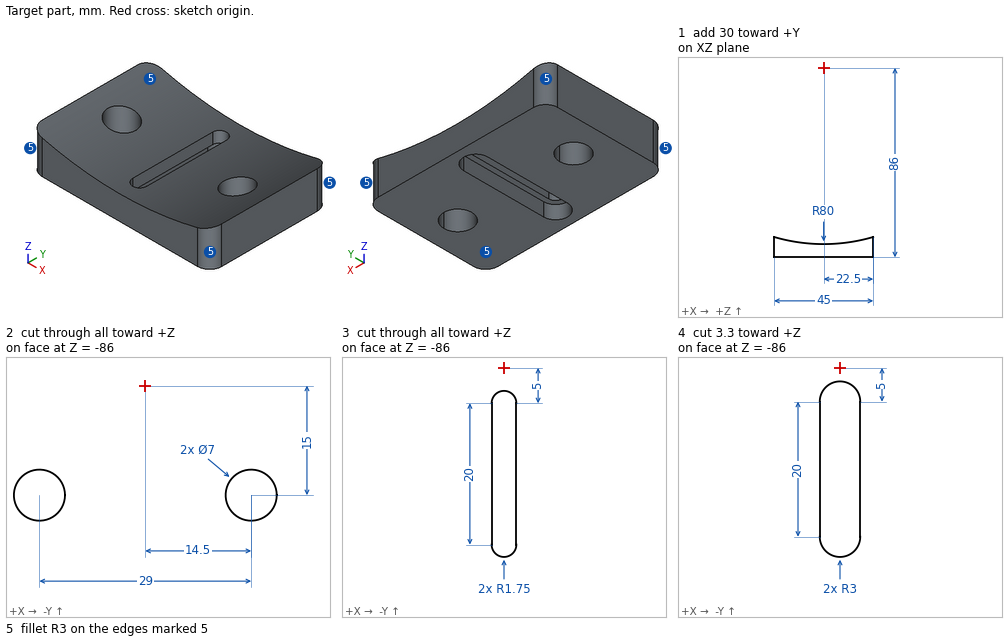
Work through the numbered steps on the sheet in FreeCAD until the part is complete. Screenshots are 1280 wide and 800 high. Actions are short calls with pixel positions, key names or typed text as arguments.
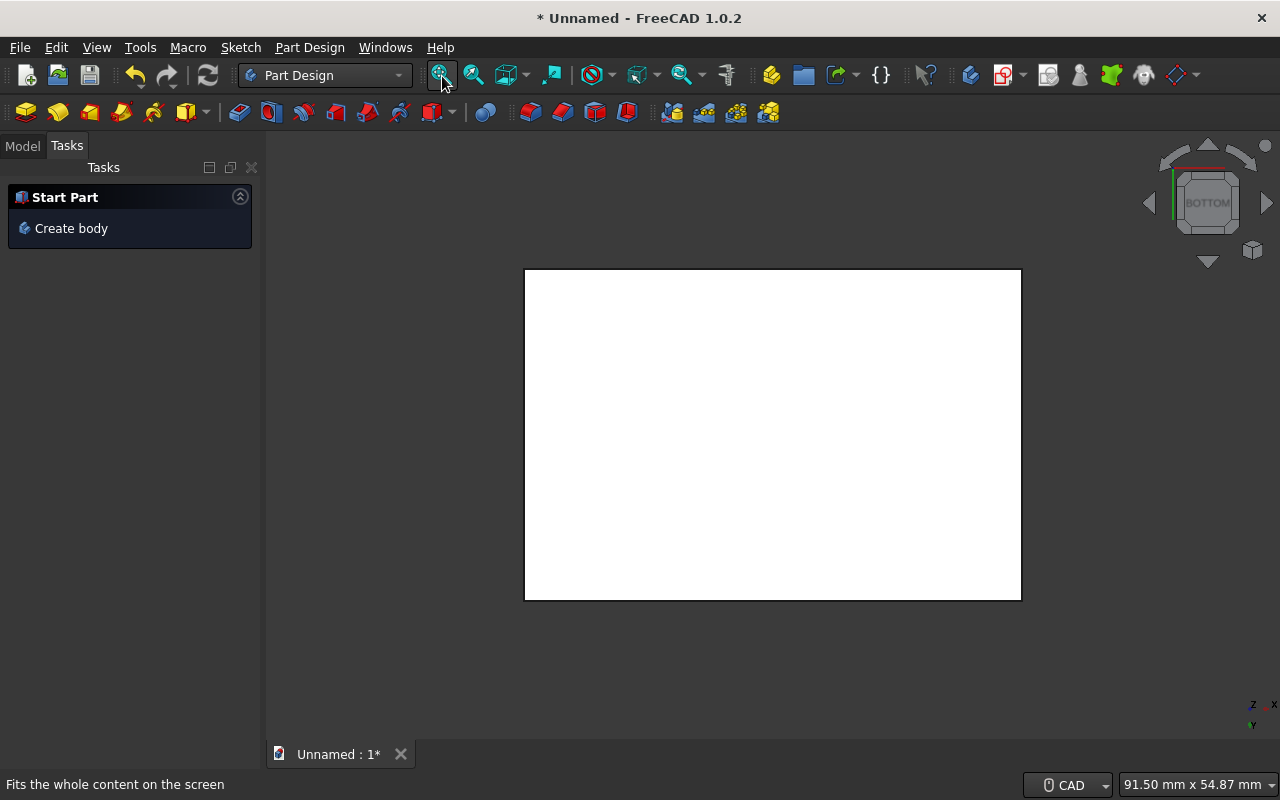
click(844, 434)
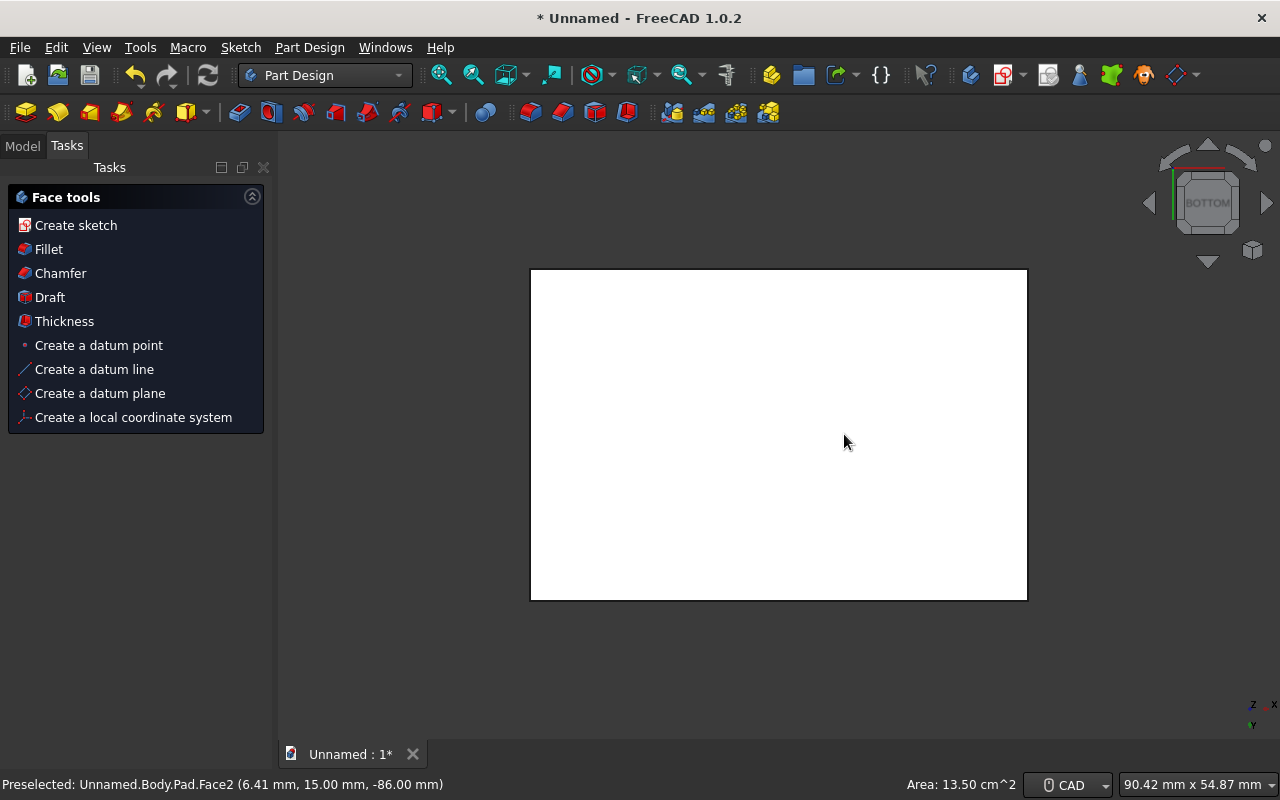
click(1004, 76)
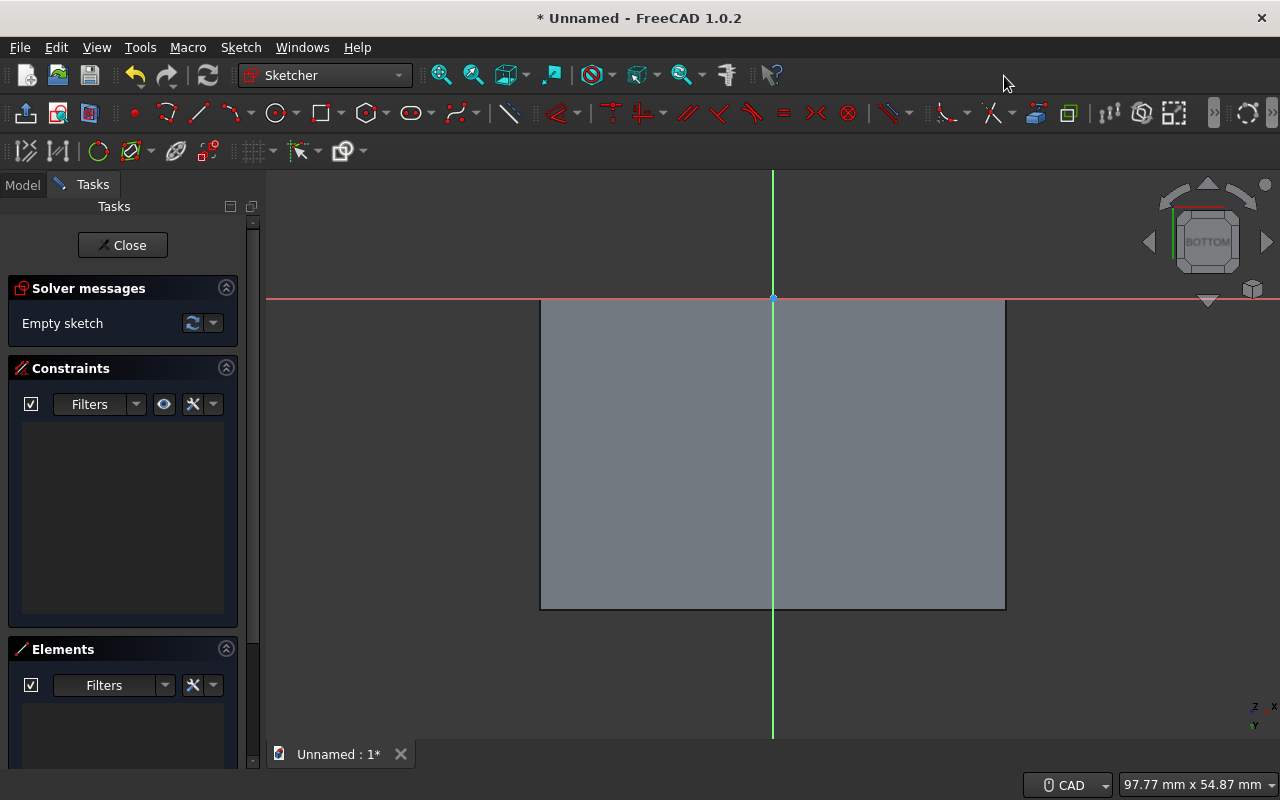
scroll(912, 274, up, 2)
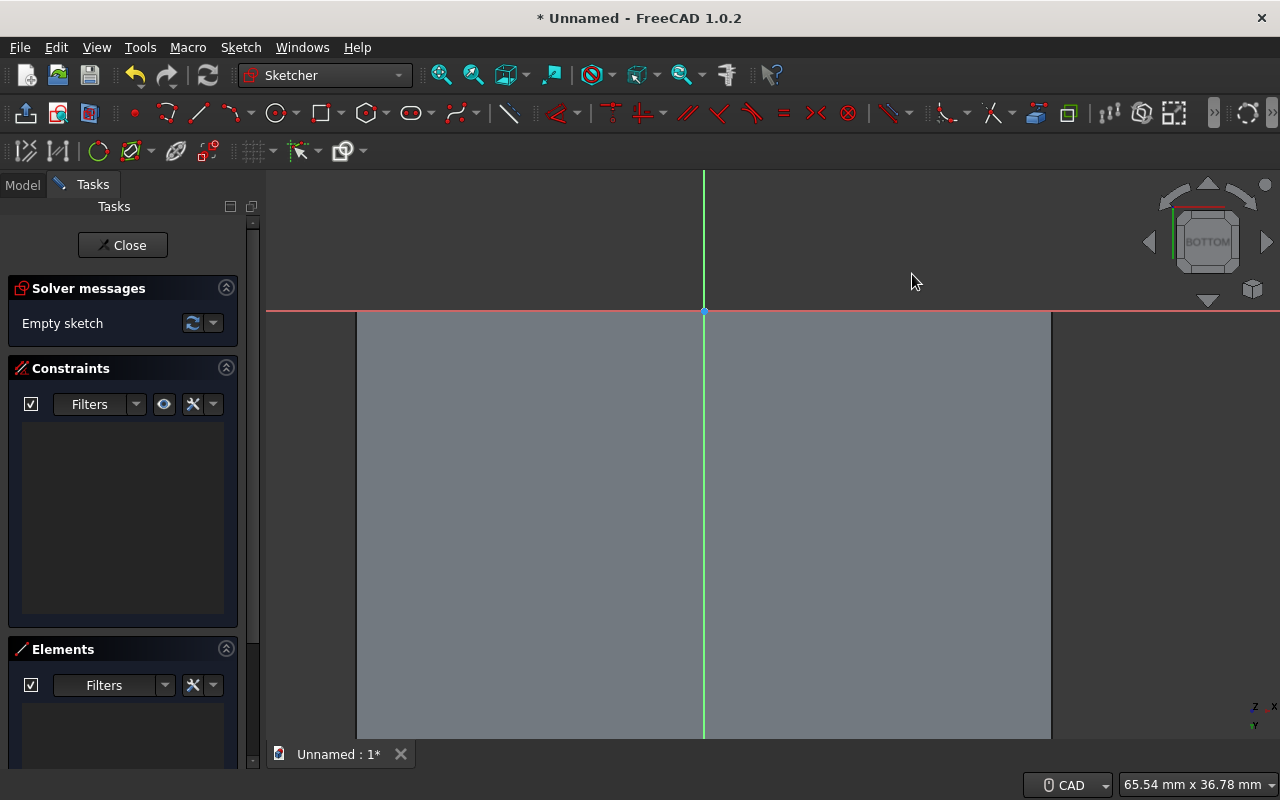
click(276, 114)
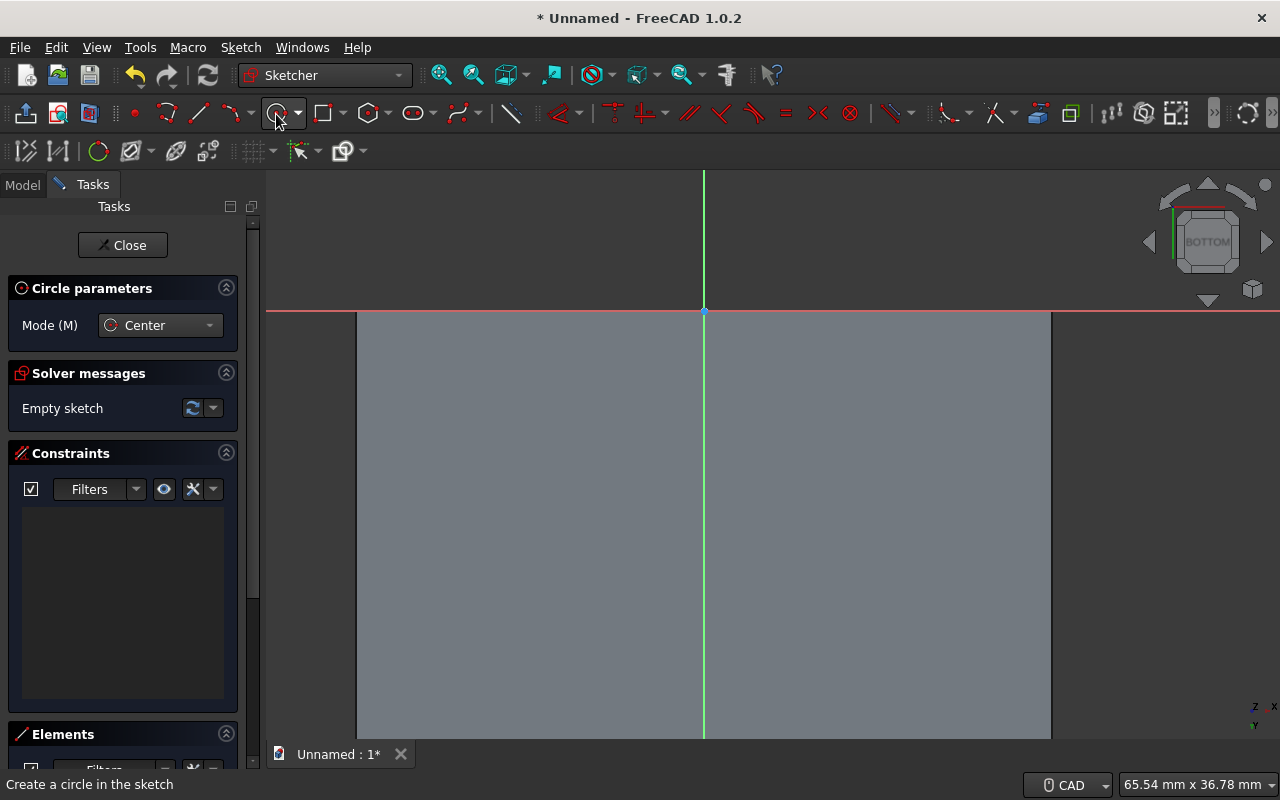
click(929, 543)
move(967, 505)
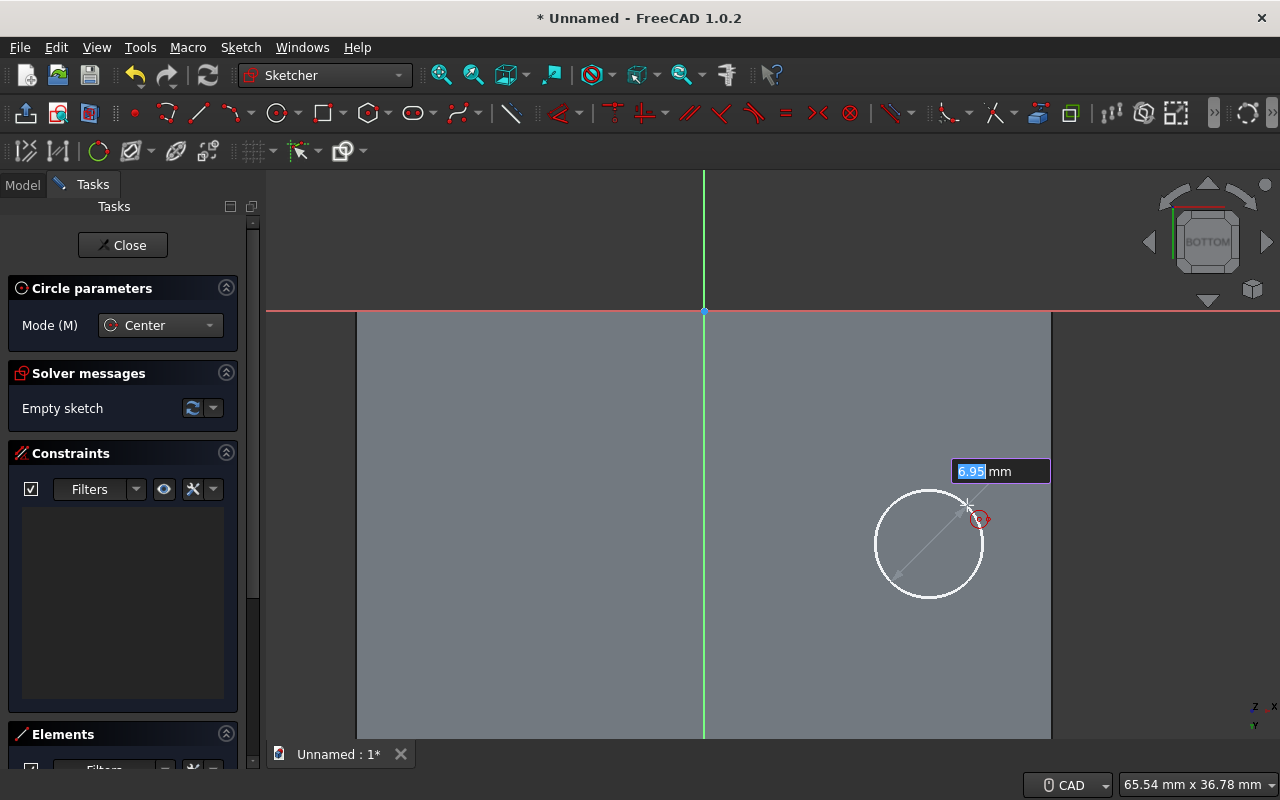
text(7)
key(Return)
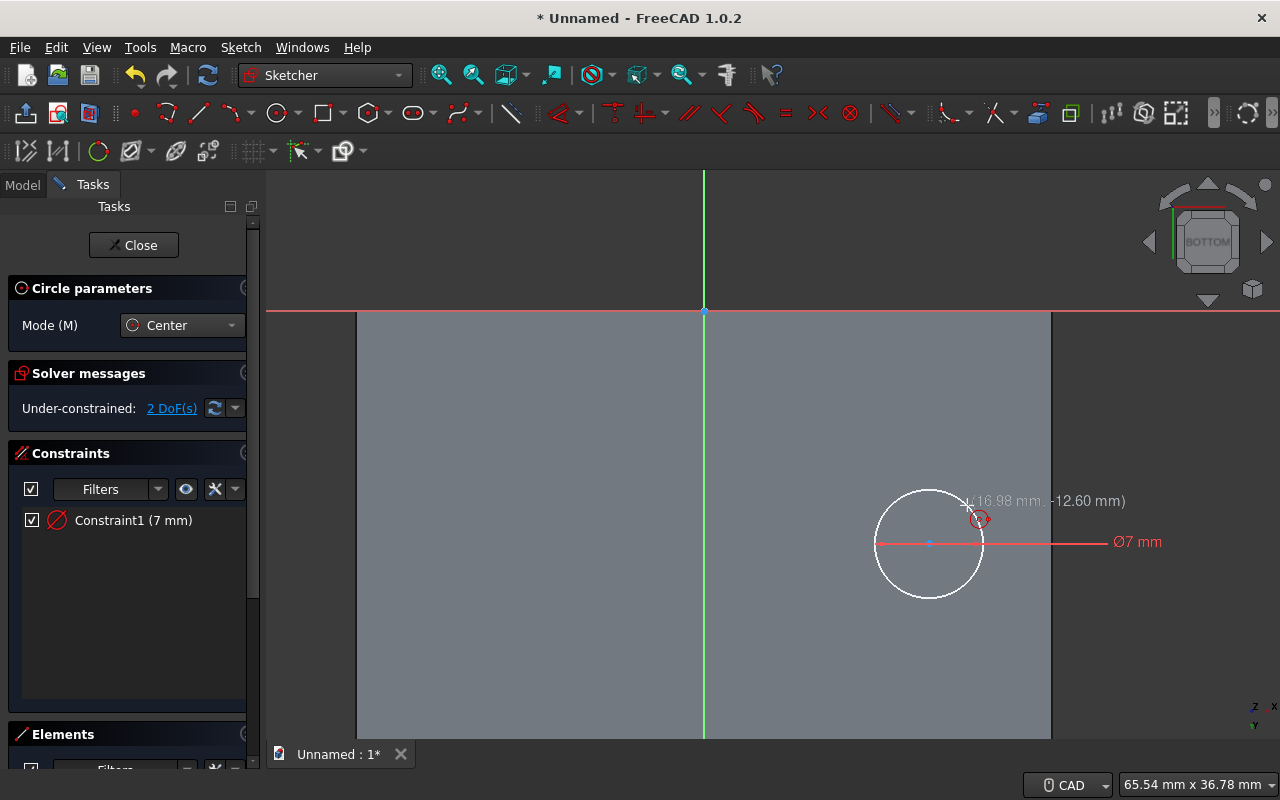
click(480, 543)
move(518, 505)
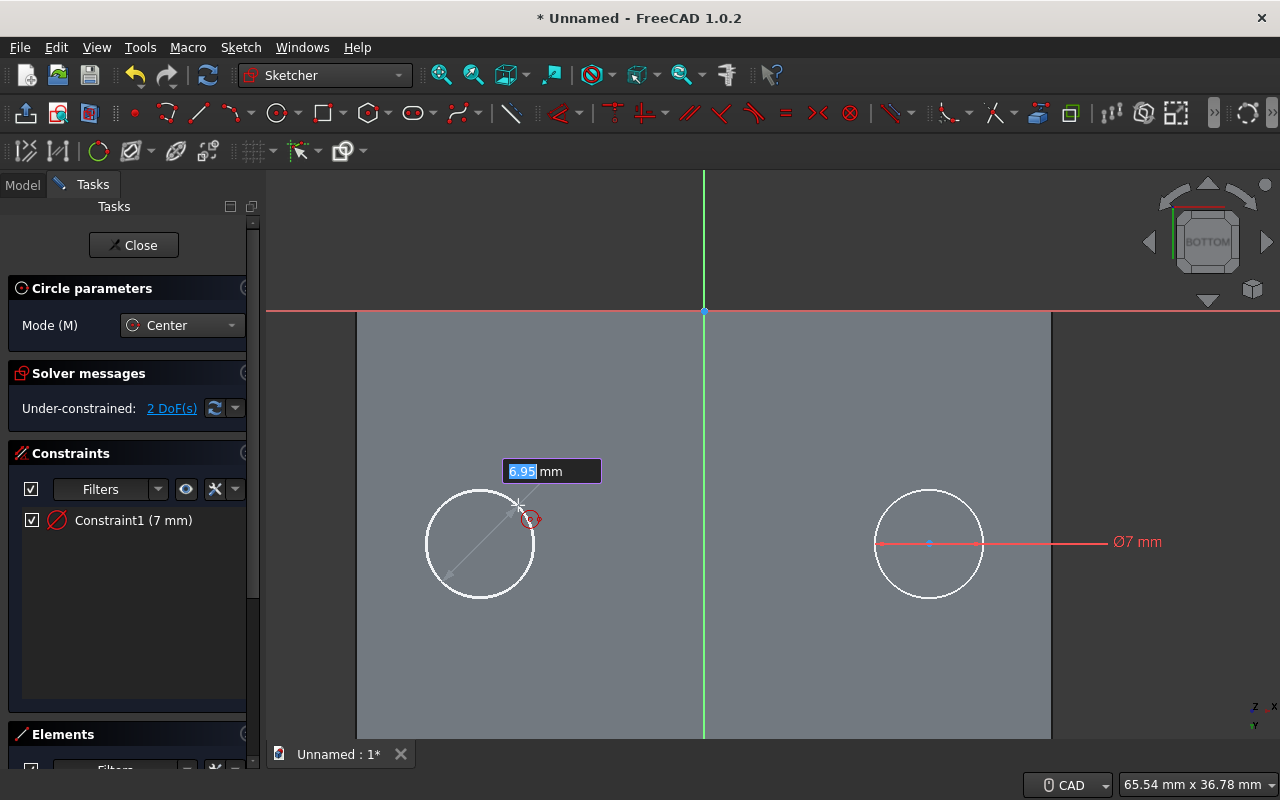
text(7)
key(Return)
key(Escape)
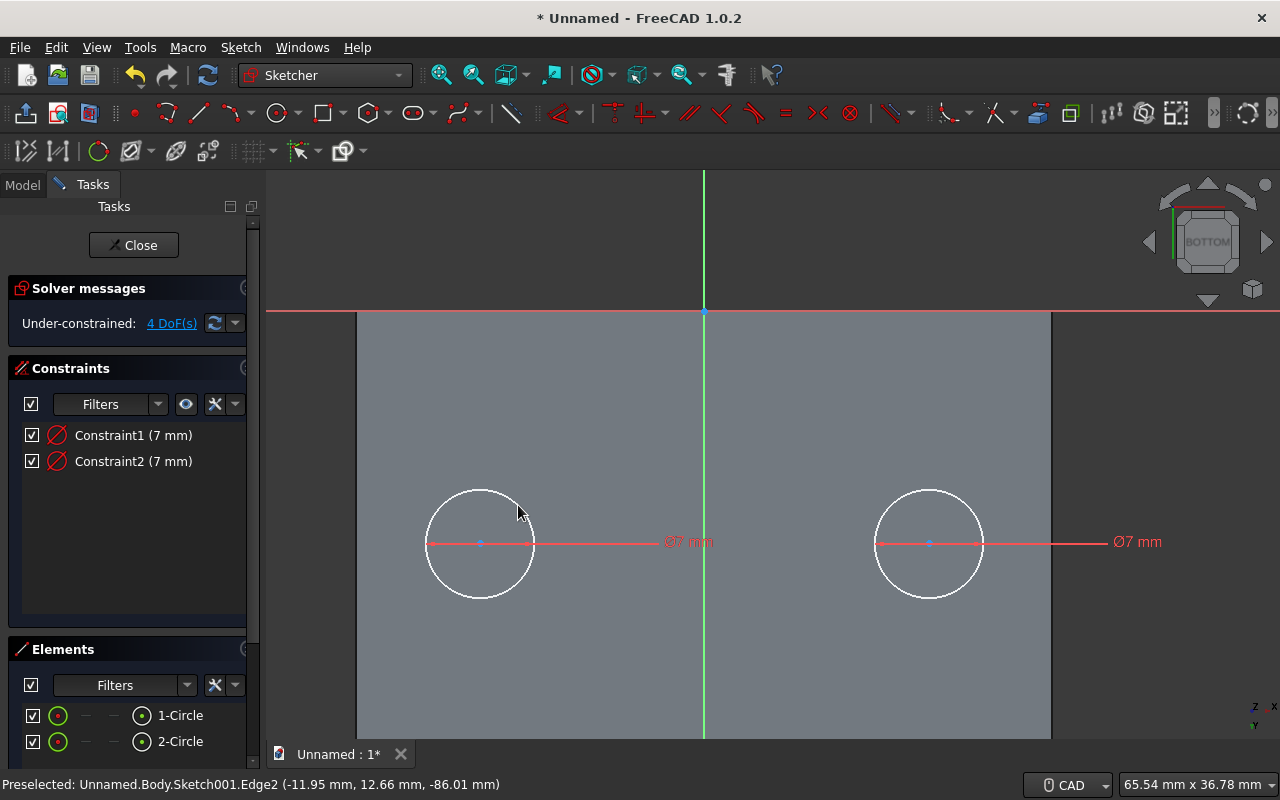
click(929, 544)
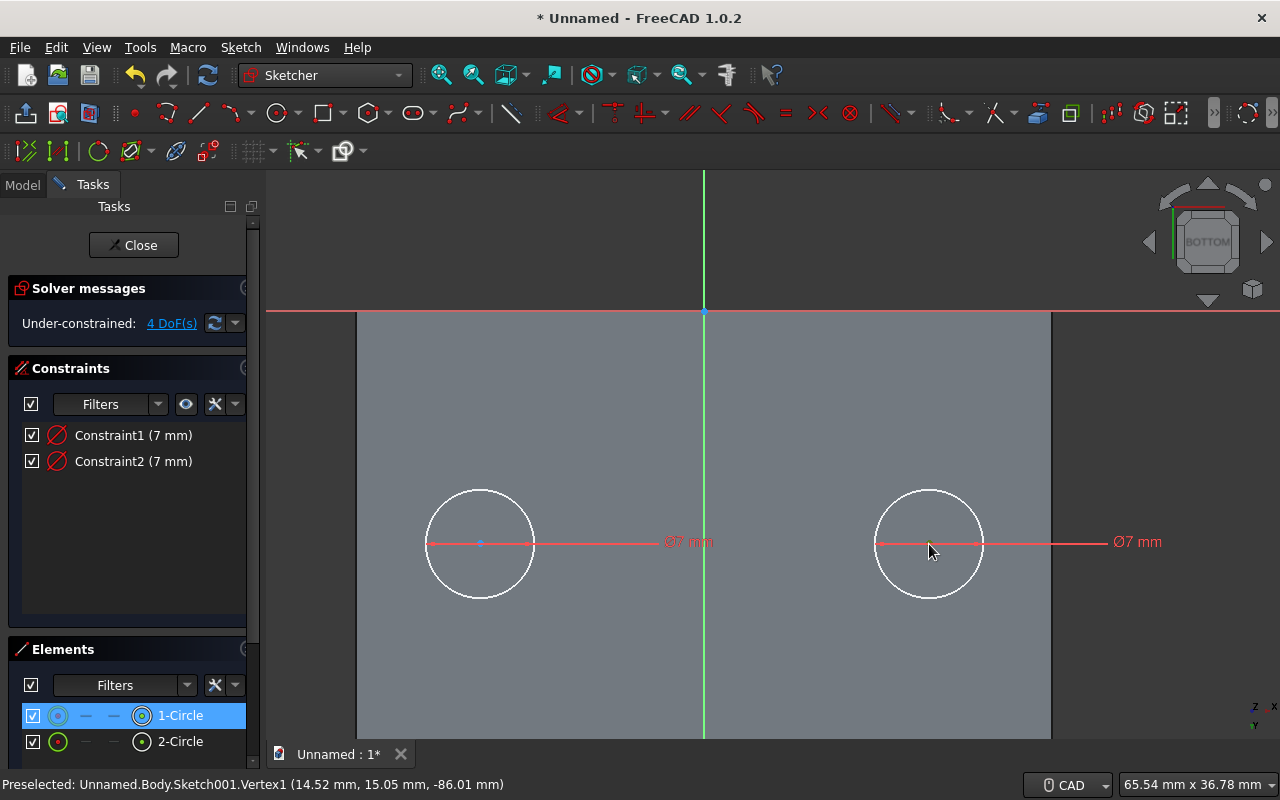
click(480, 544)